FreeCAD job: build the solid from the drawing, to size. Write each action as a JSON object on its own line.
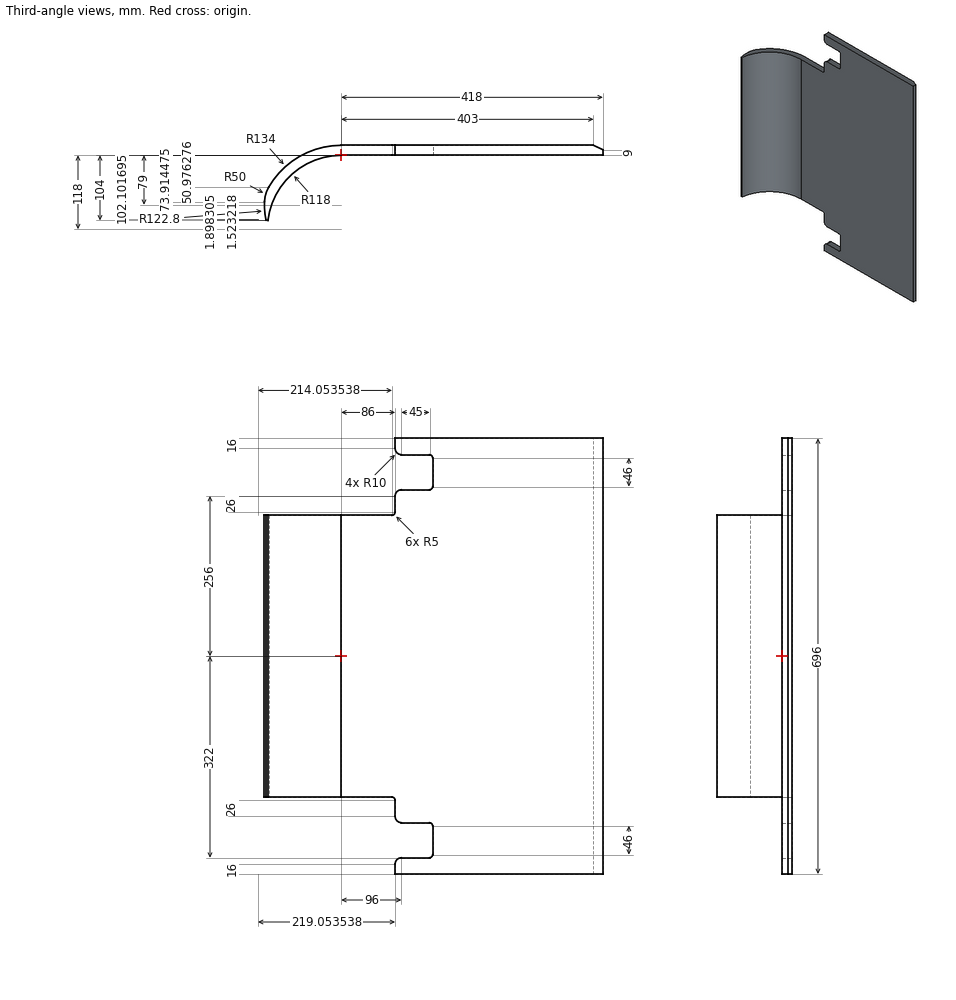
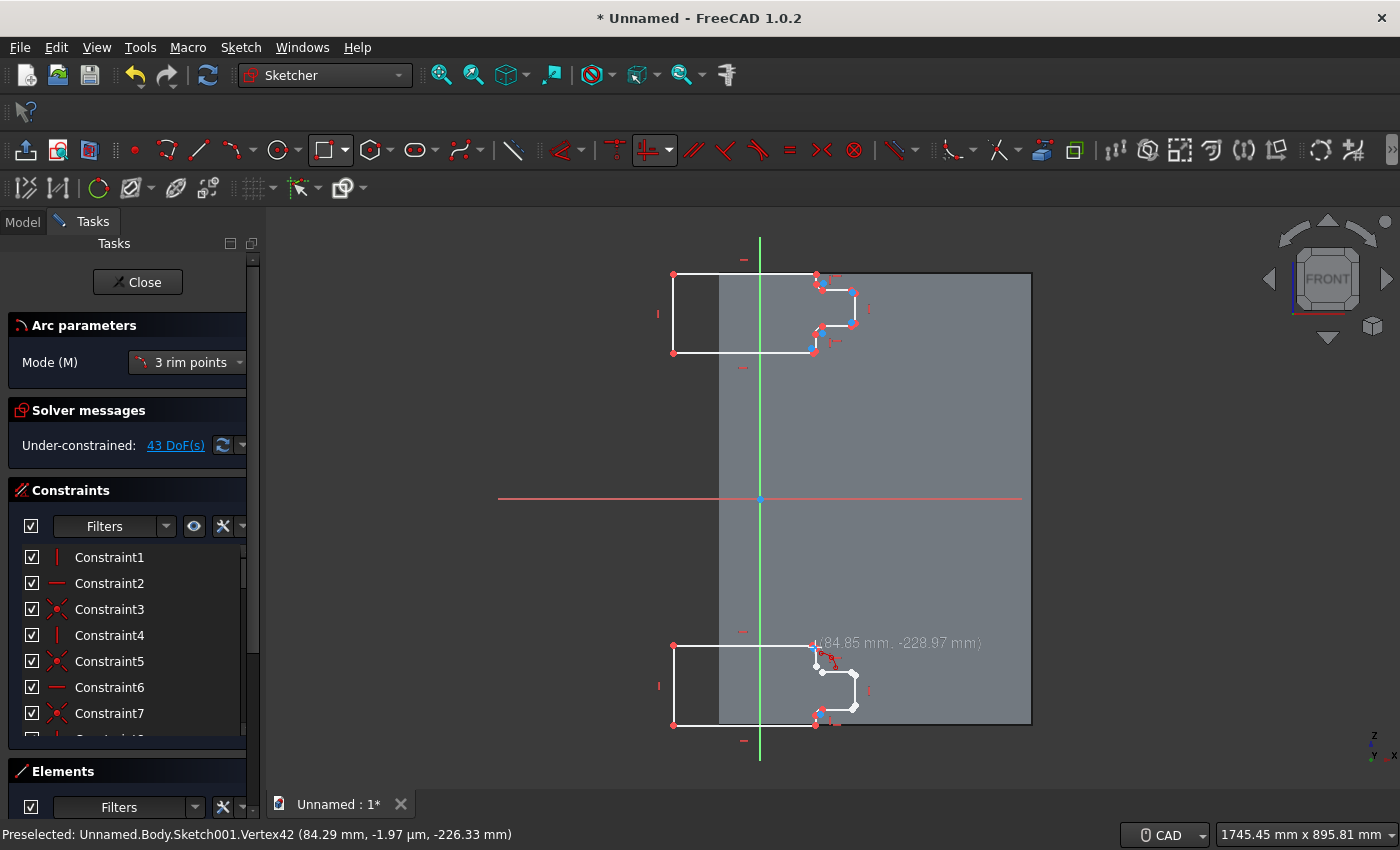
{"action": "scroll", "coordinate": [816, 665], "scroll_direction": "up", "scroll_amount": 4}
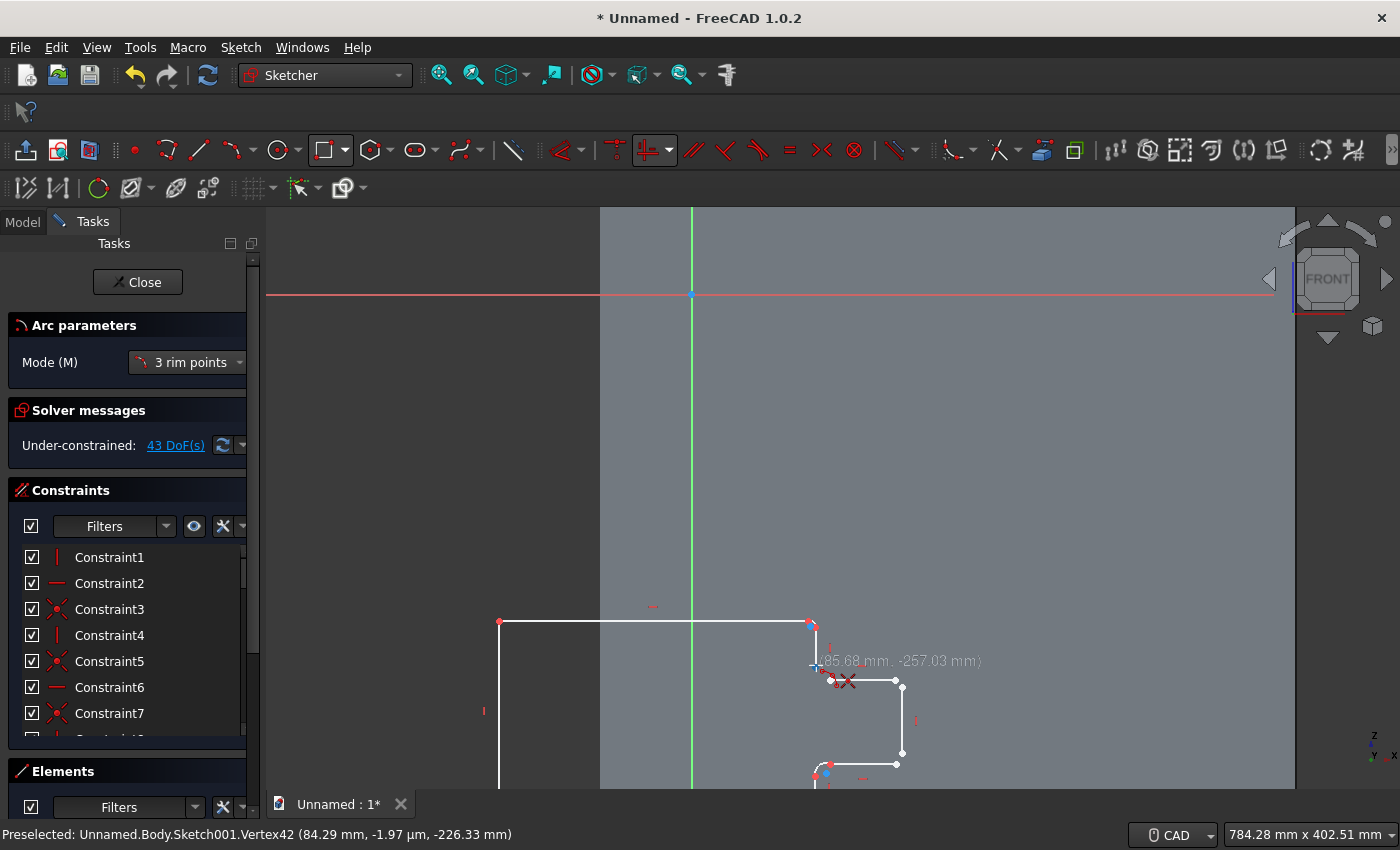
{"action": "left_click", "coordinate": [816, 667]}
{"action": "left_click", "coordinate": [830, 680]}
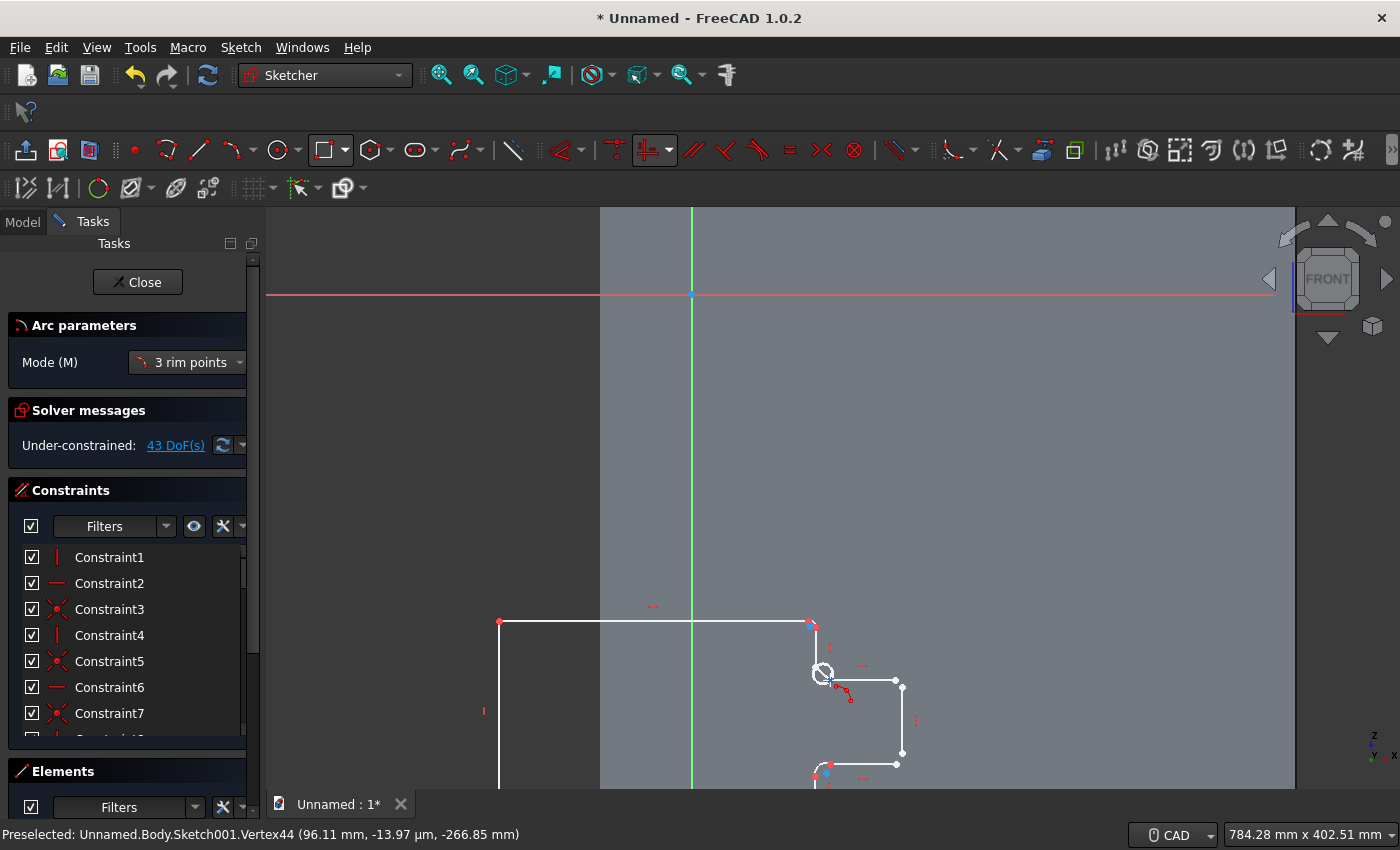
{"action": "scroll", "coordinate": [820, 675], "scroll_direction": "up", "scroll_amount": 7}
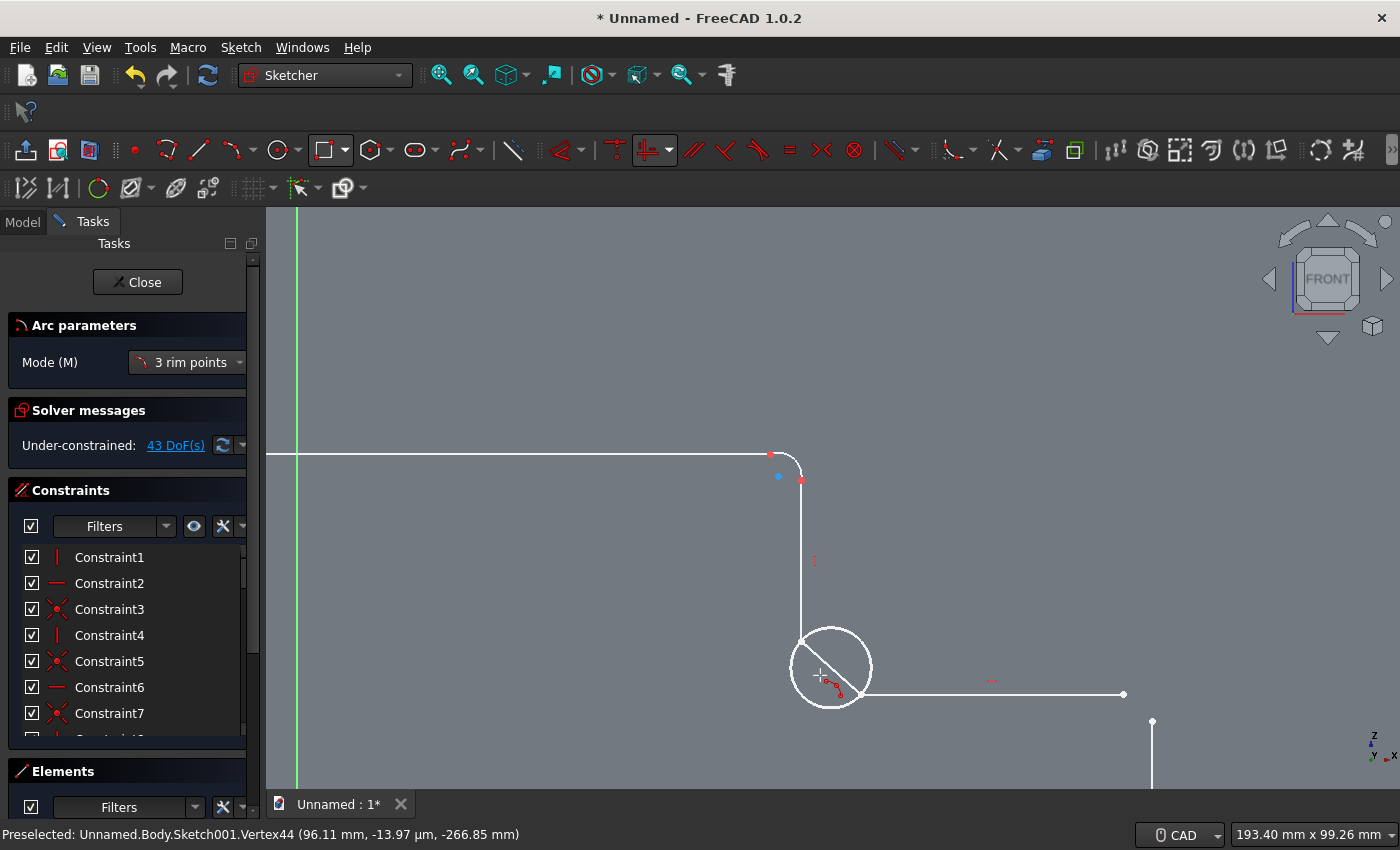
{"action": "left_click", "coordinate": [819, 672]}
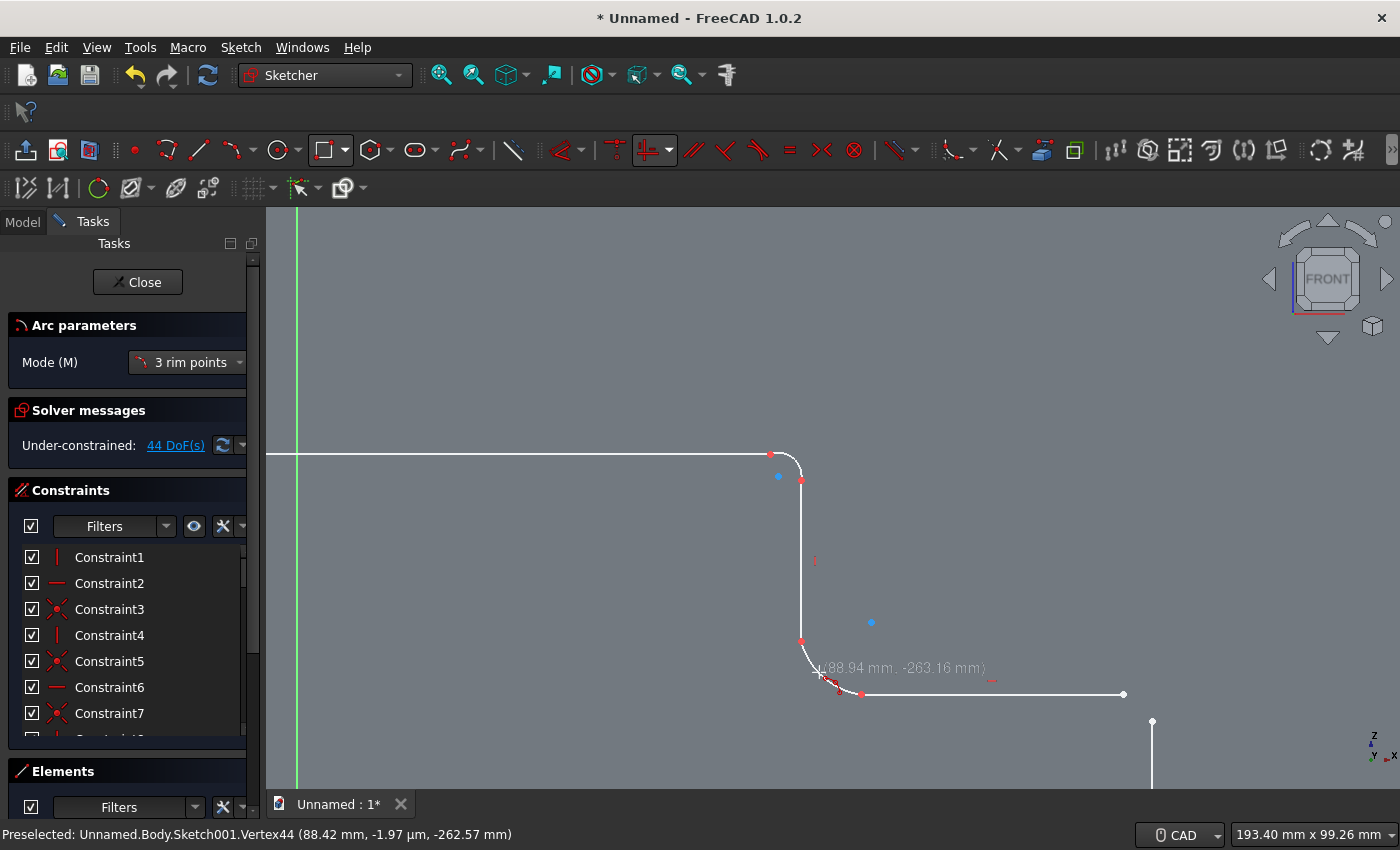
{"action": "left_click", "coordinate": [1124, 695]}
{"action": "left_click", "coordinate": [1152, 721]}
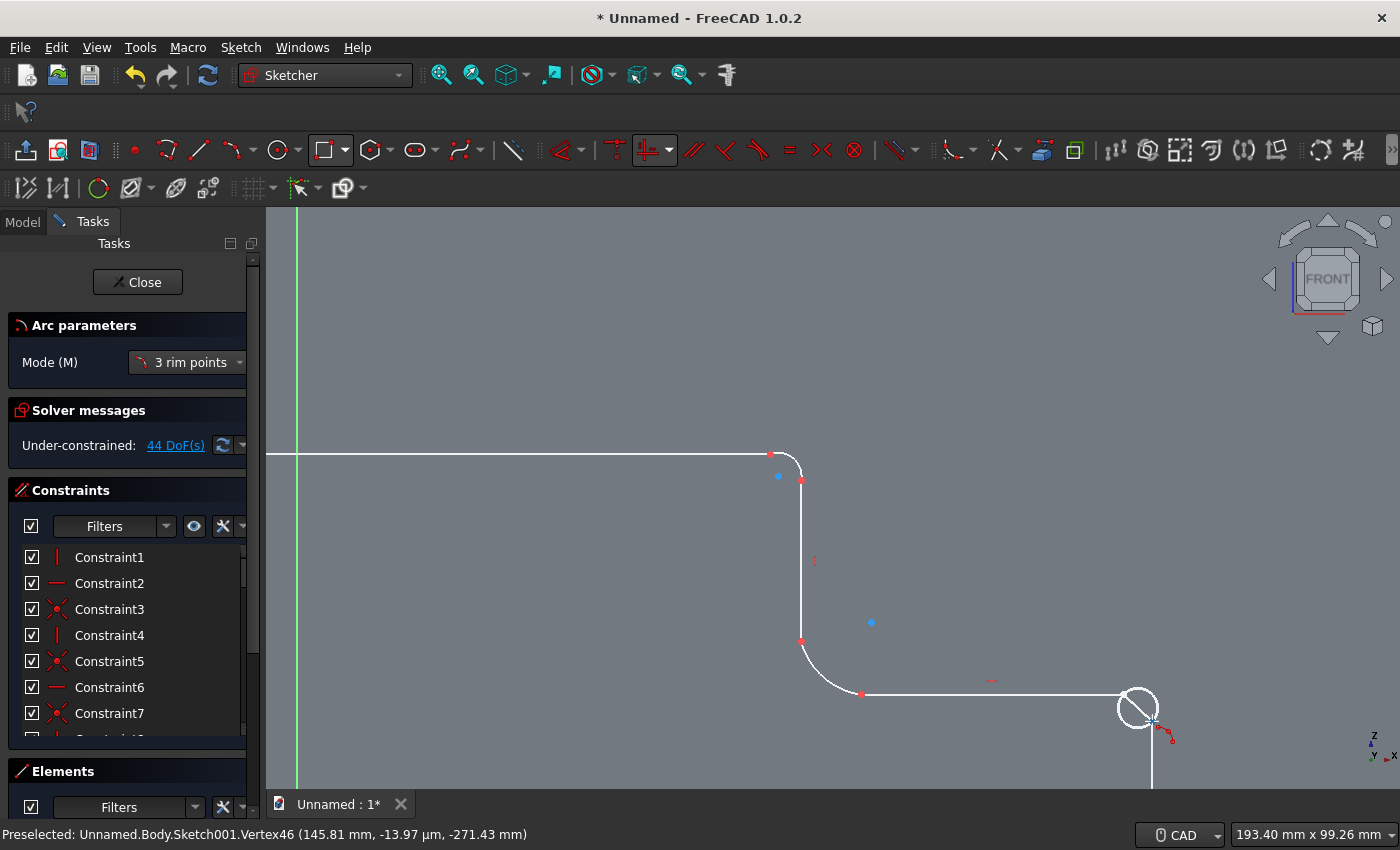
{"action": "scroll", "coordinate": [1145, 698], "scroll_direction": "up", "scroll_amount": 4}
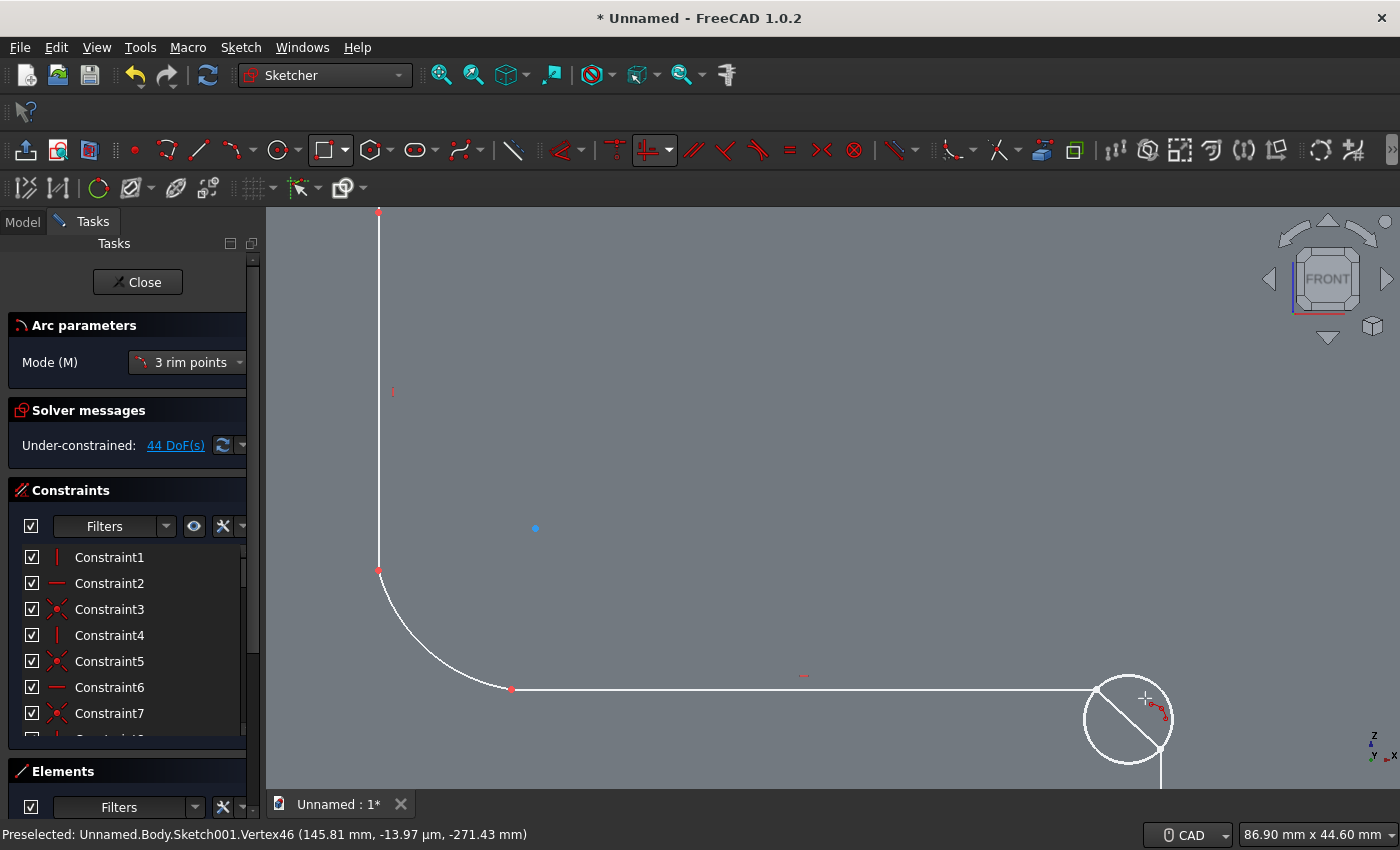
{"action": "left_click", "coordinate": [1144, 698]}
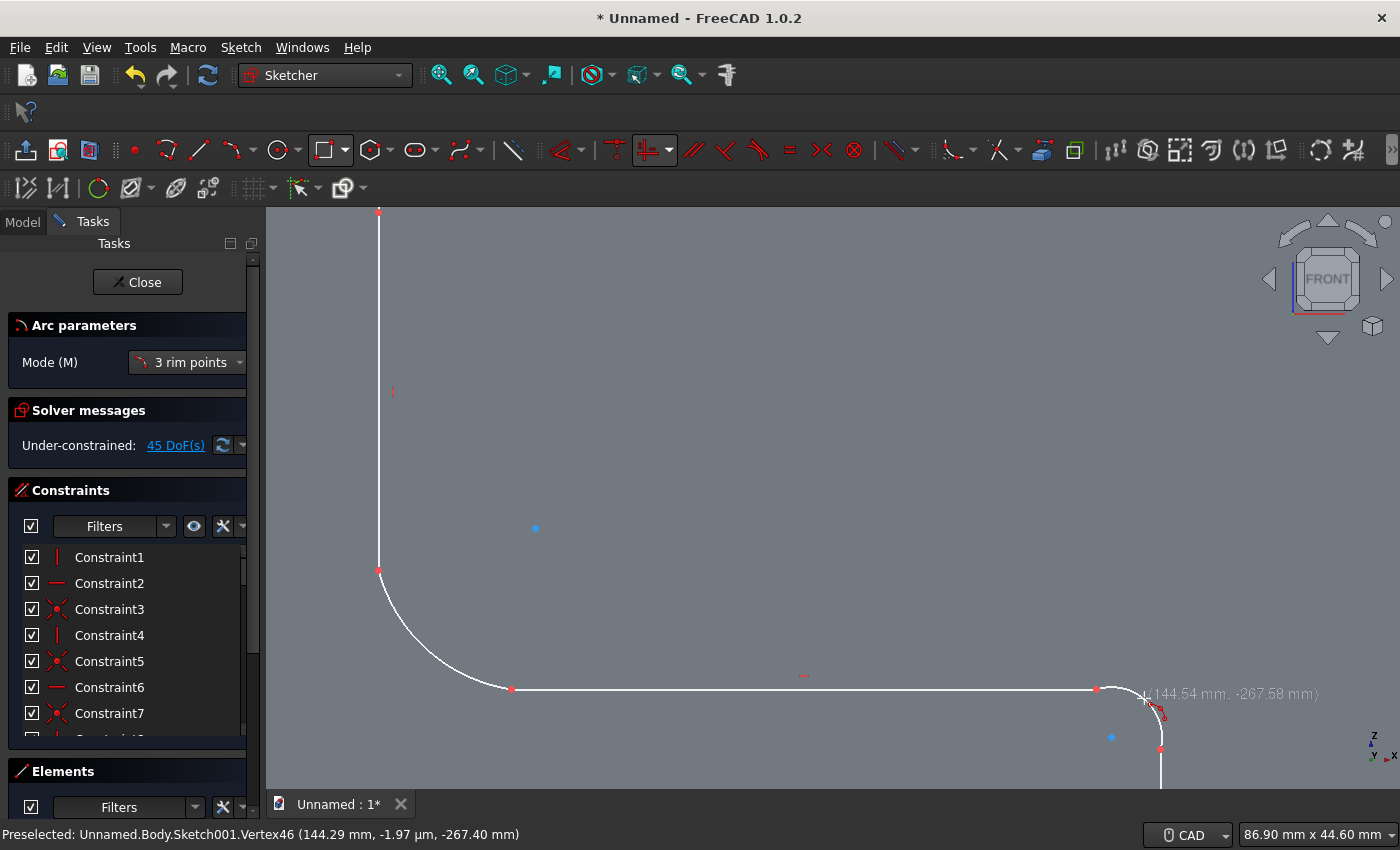
{"action": "scroll", "coordinate": [839, 670], "scroll_direction": "down", "scroll_amount": 15}